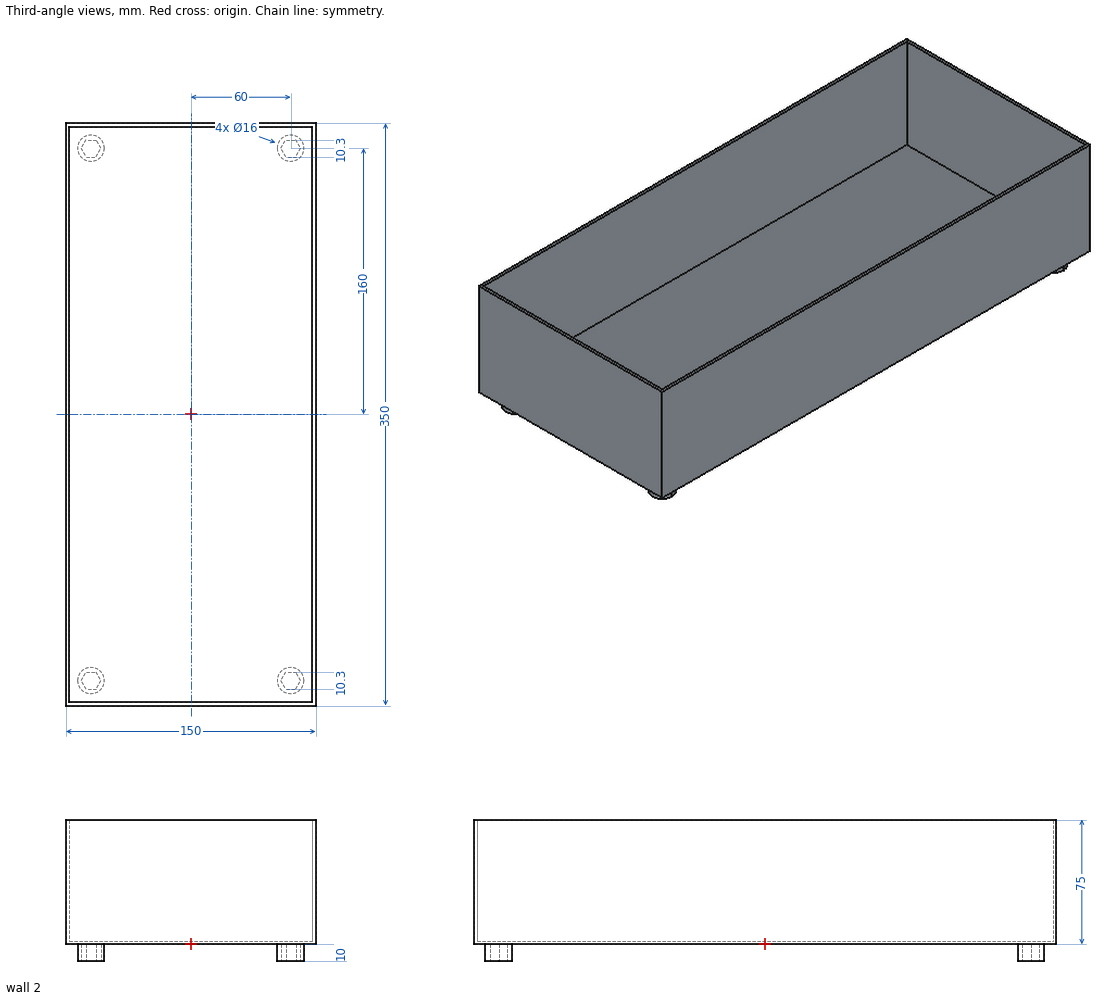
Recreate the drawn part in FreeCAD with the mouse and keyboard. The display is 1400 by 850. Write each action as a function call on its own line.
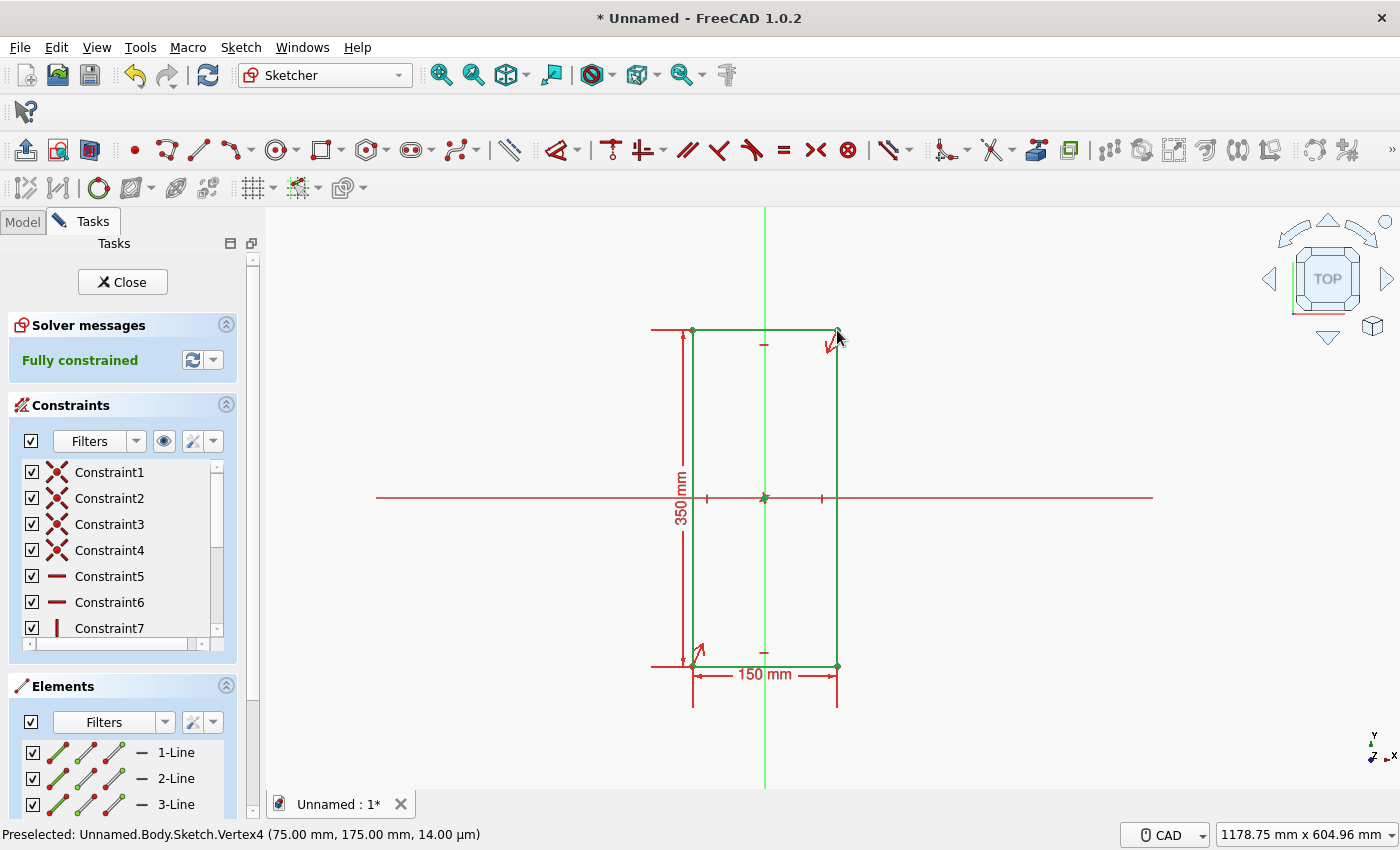
click(123, 282)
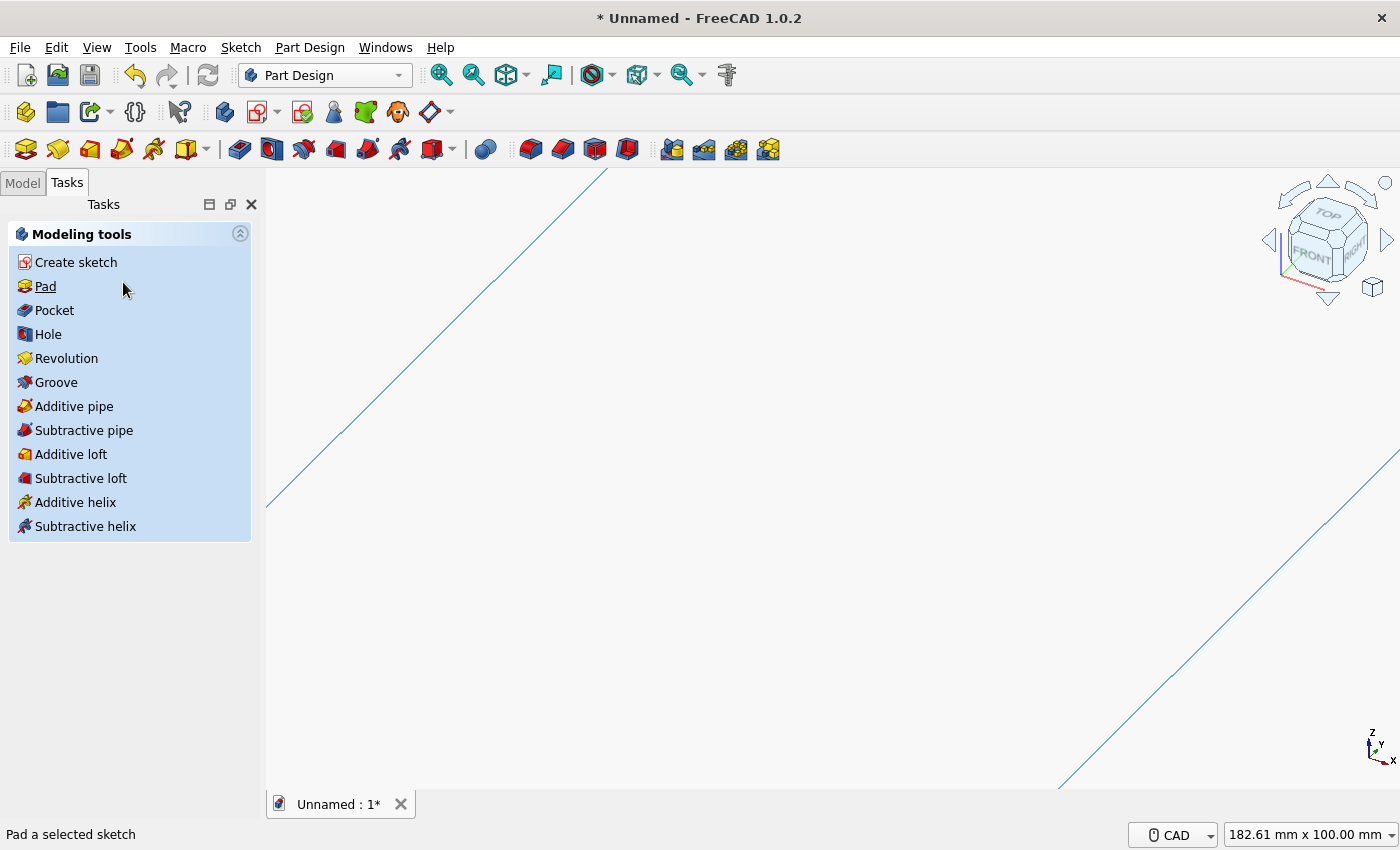
click(26, 150)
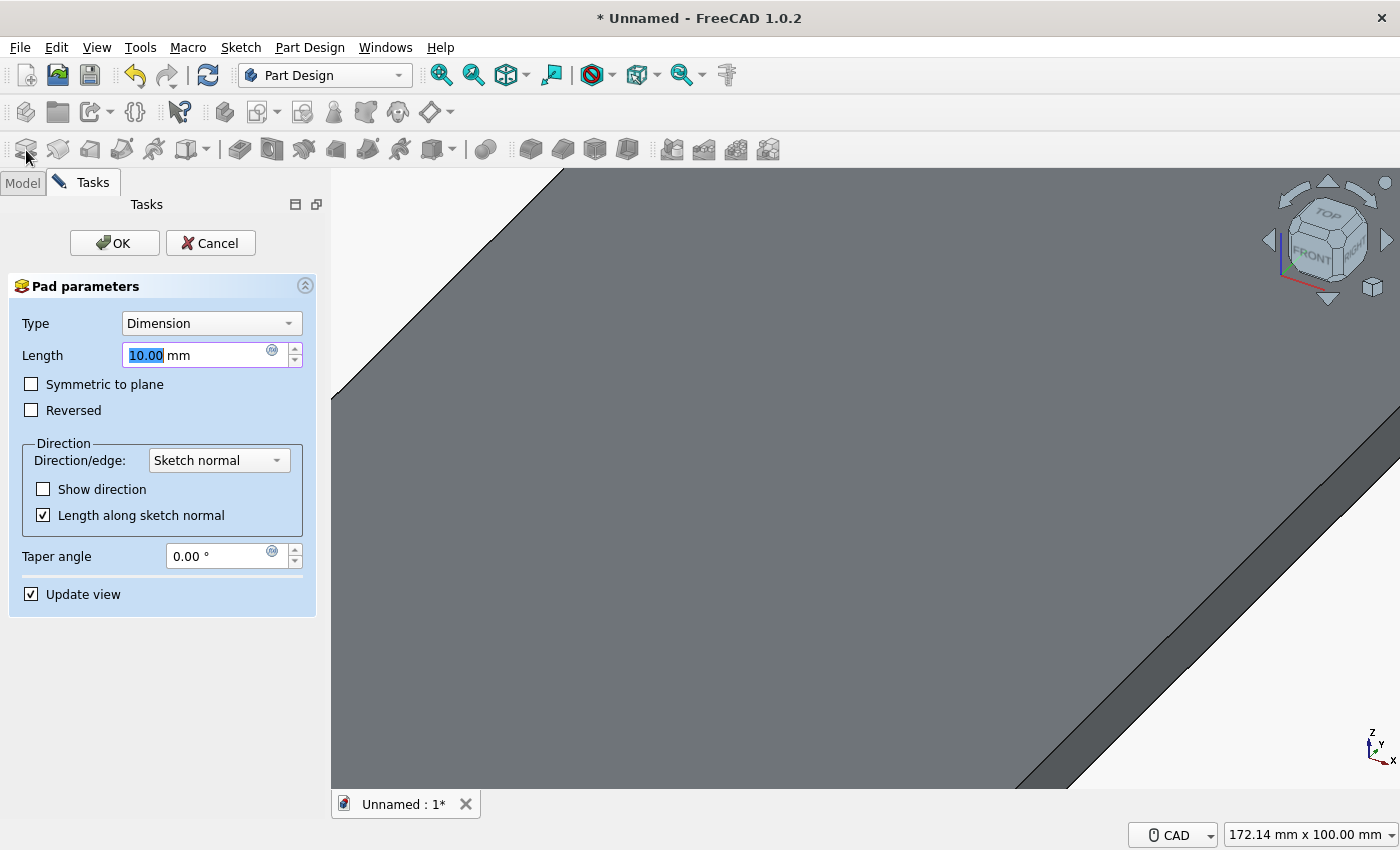
text(75)
key(Tab)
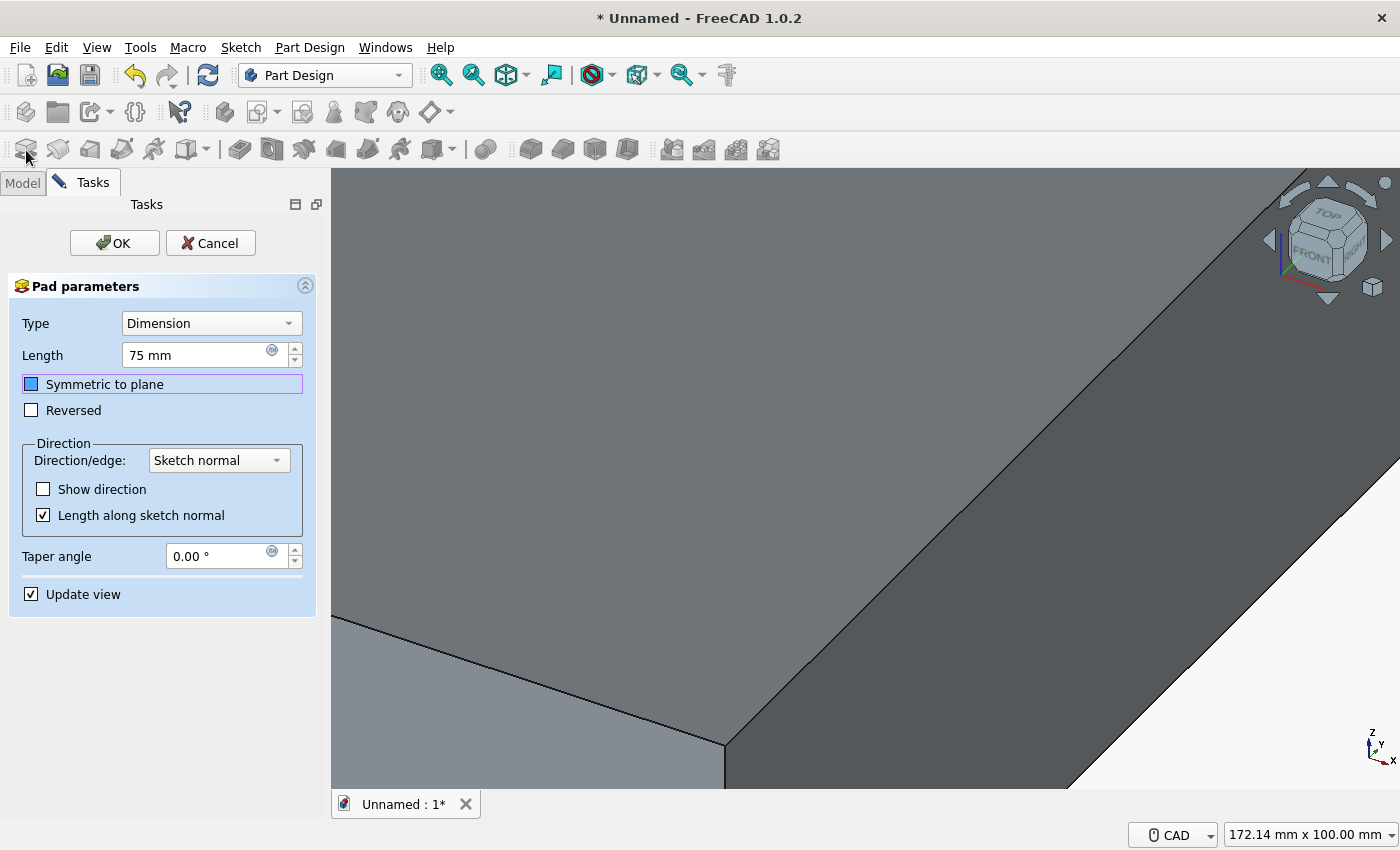
click(115, 243)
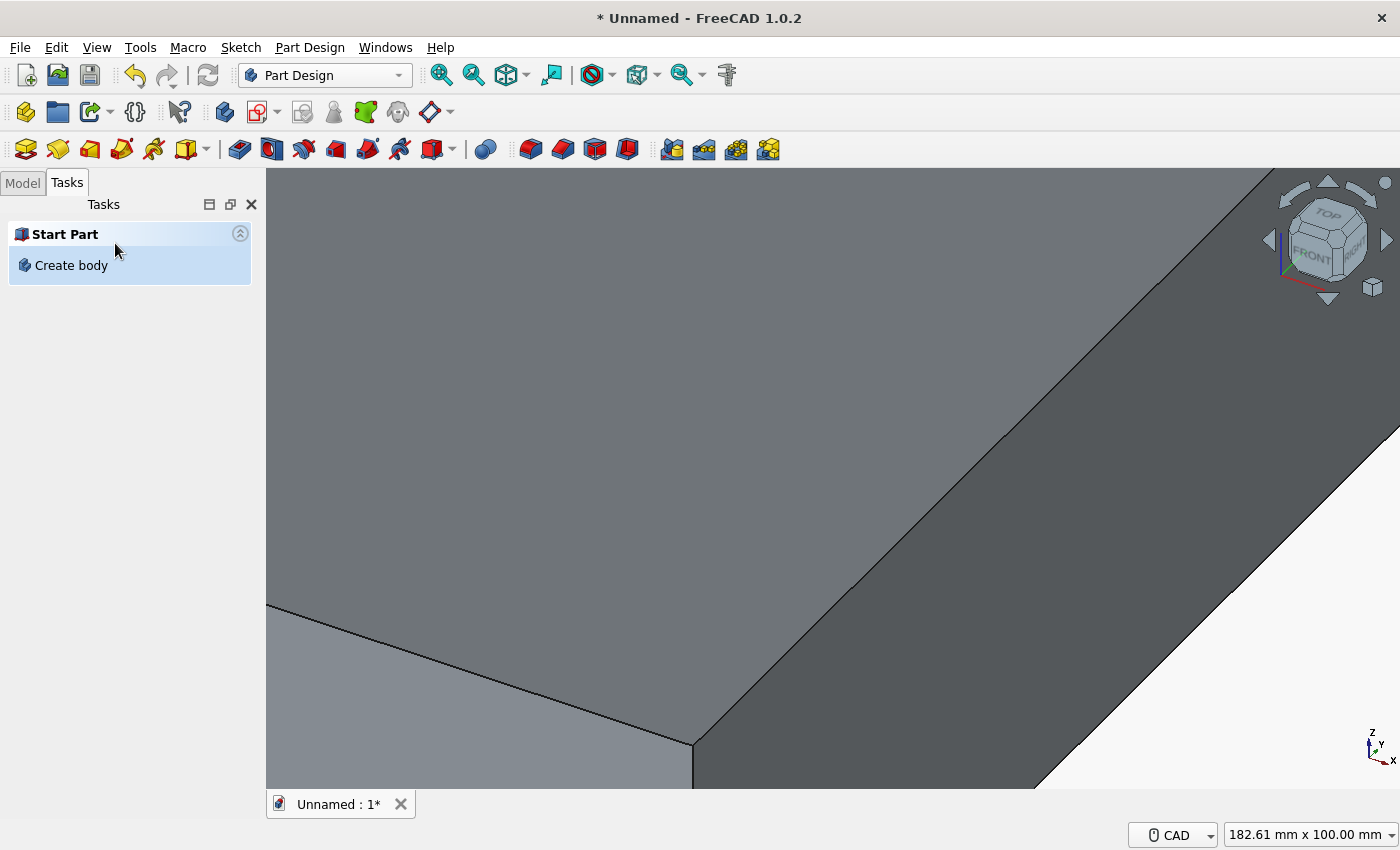
click(442, 76)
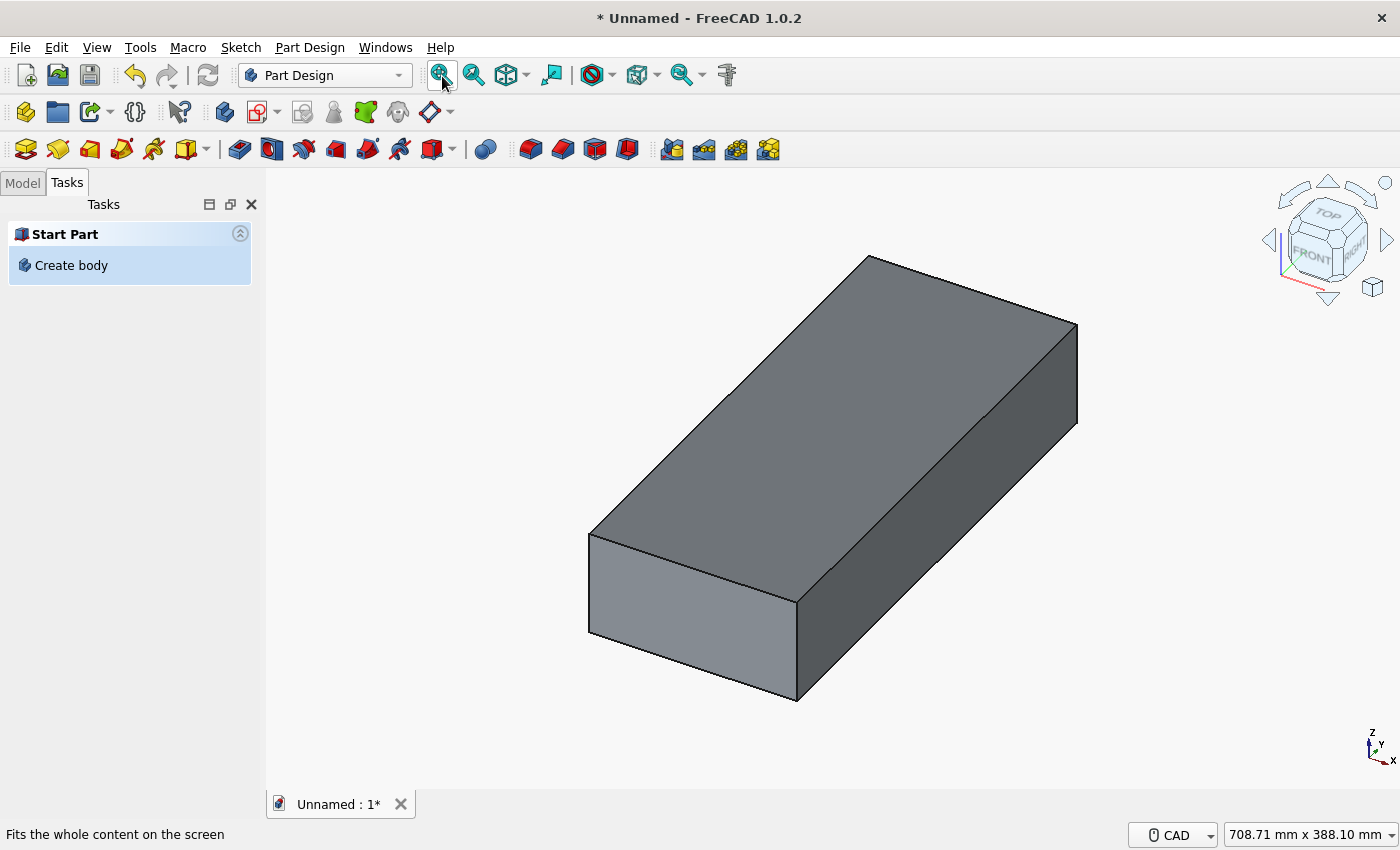
click(913, 349)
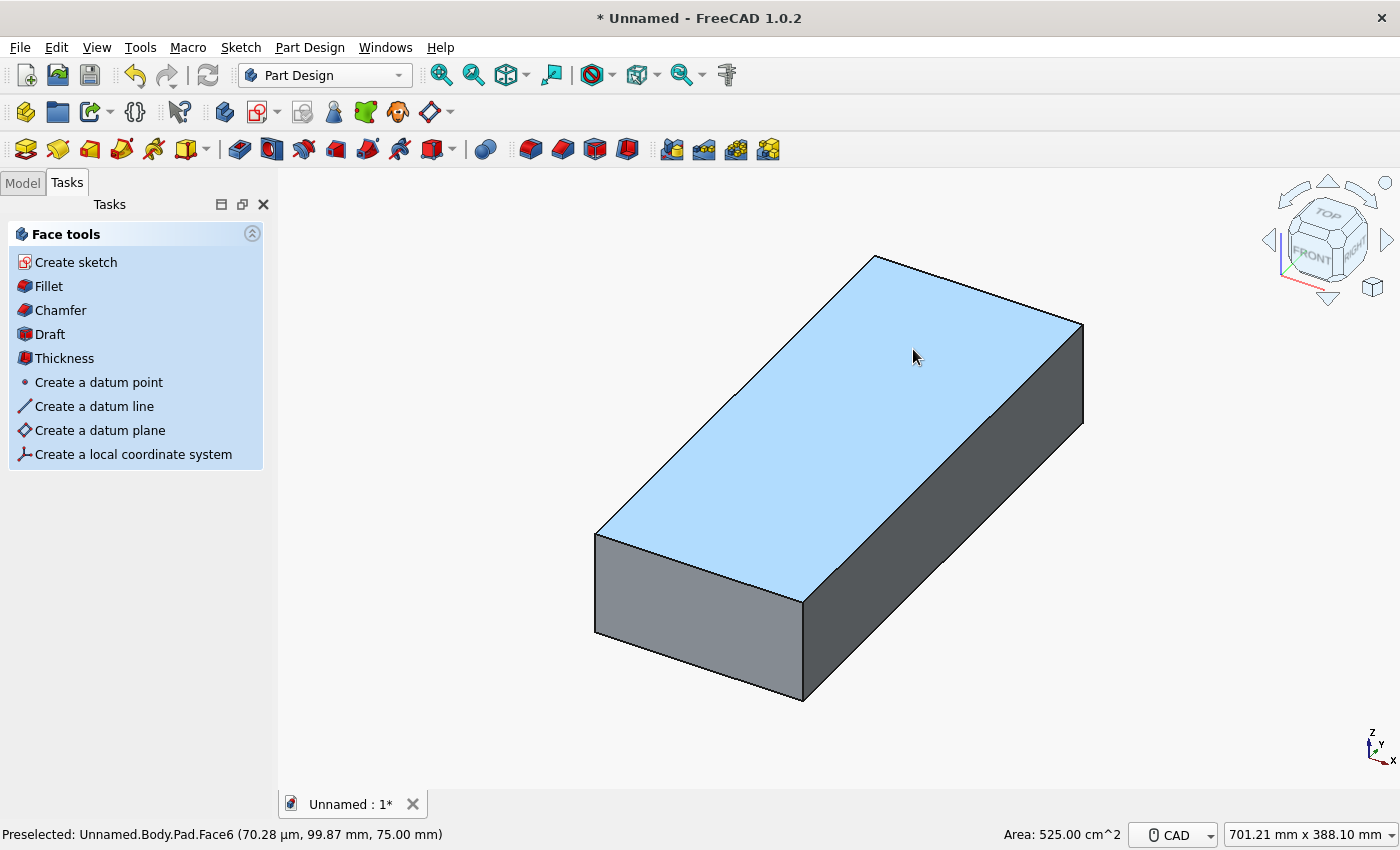
click(628, 150)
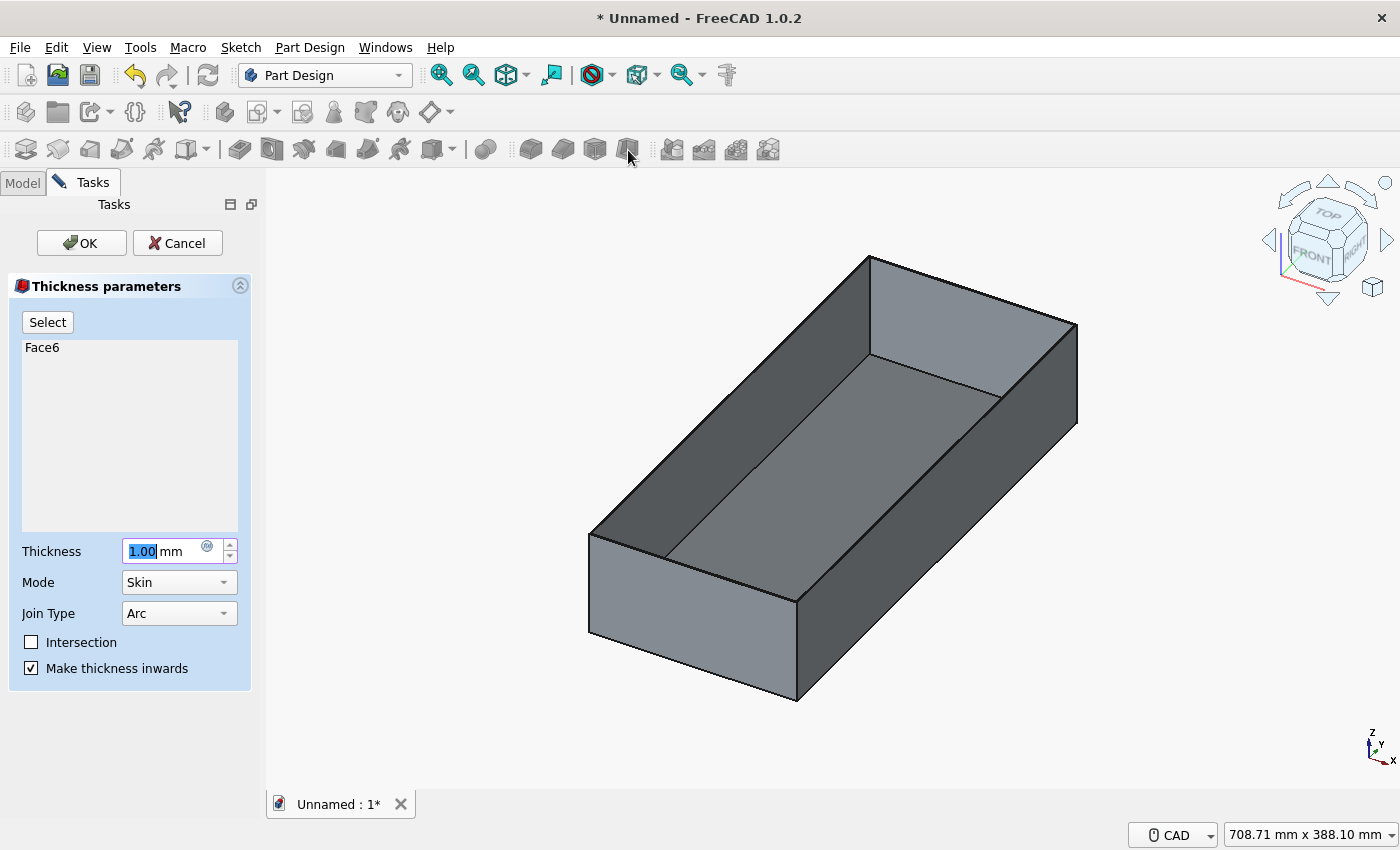
text(2)
key(Tab)